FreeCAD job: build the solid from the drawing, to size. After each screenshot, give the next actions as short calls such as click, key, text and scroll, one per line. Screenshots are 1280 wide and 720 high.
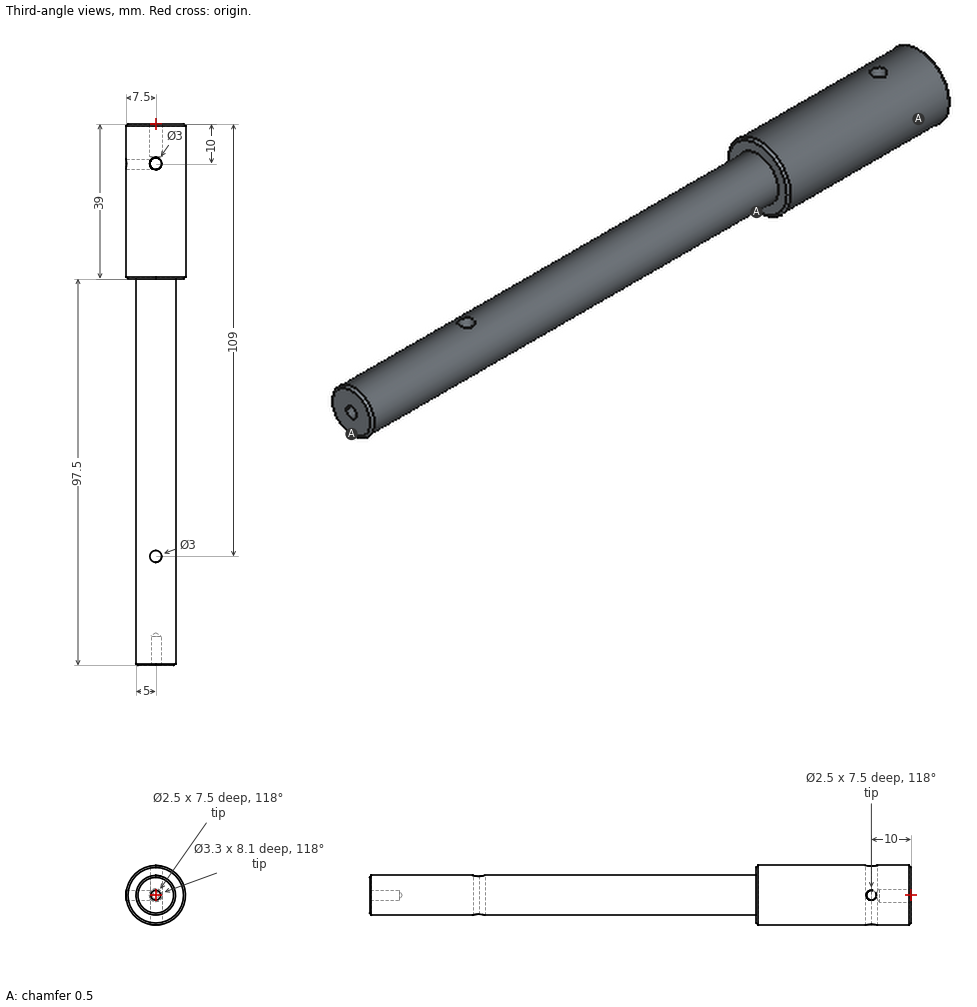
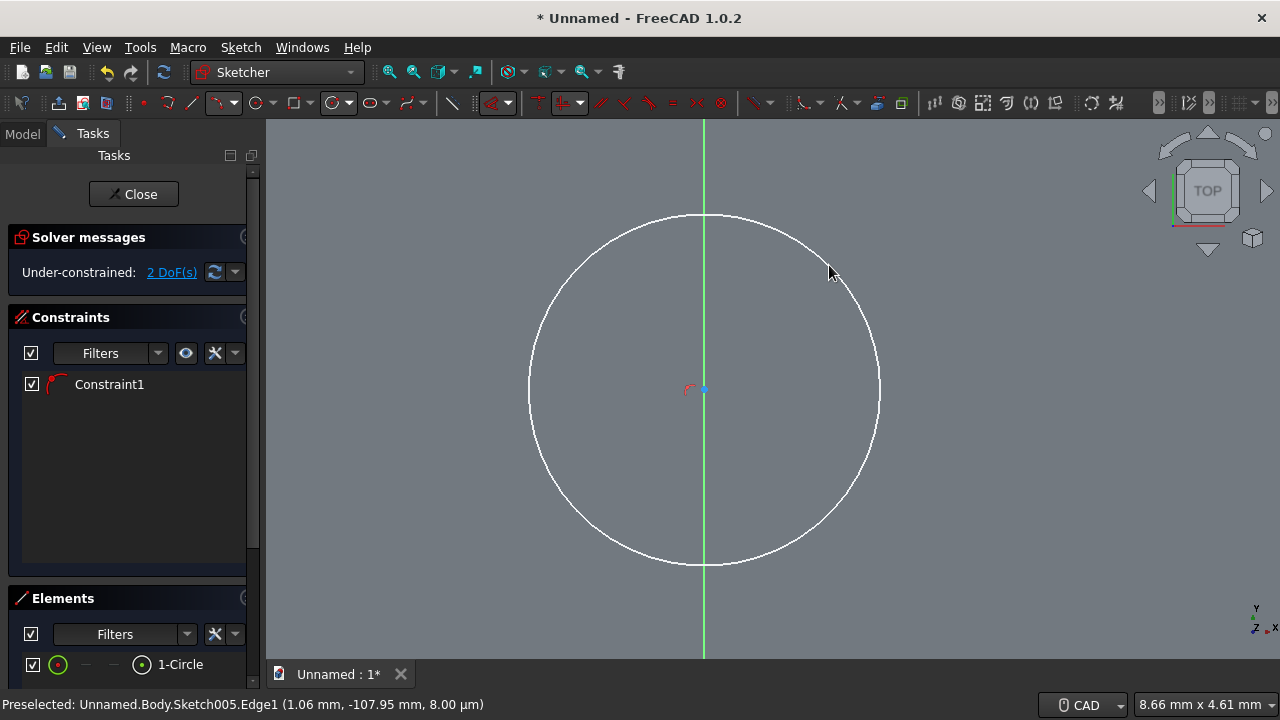
click(828, 265)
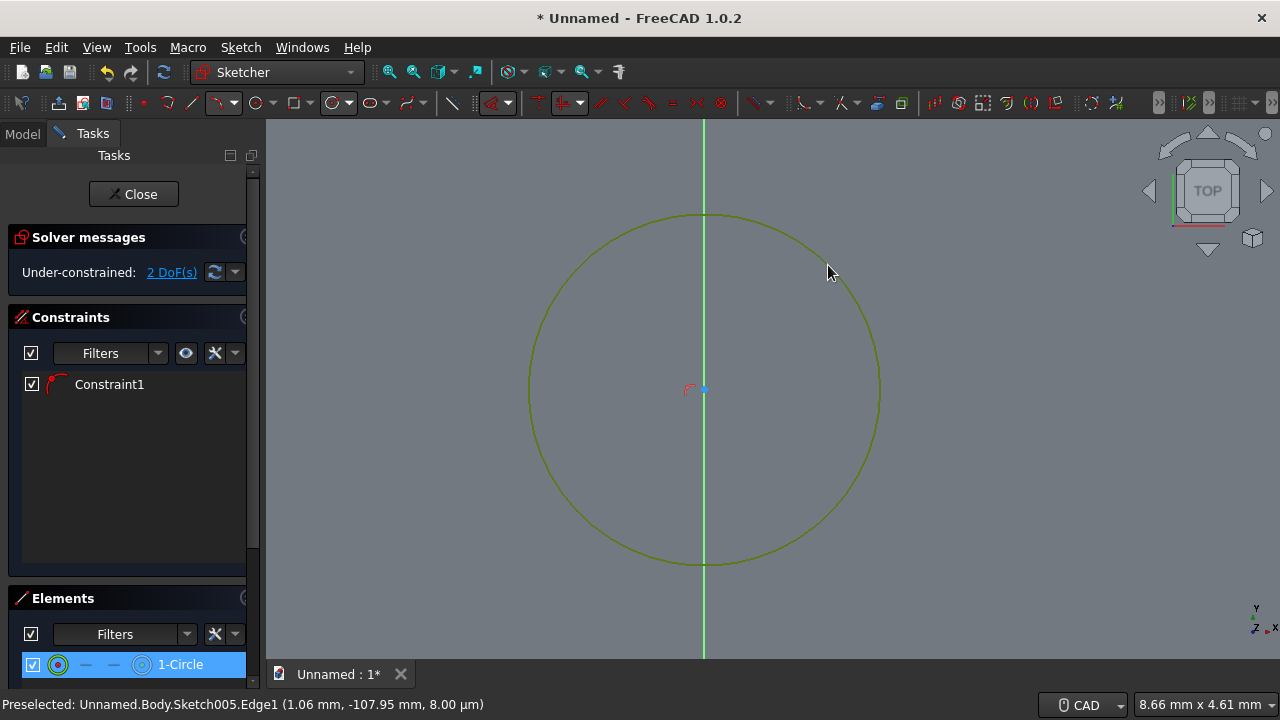
click(510, 104)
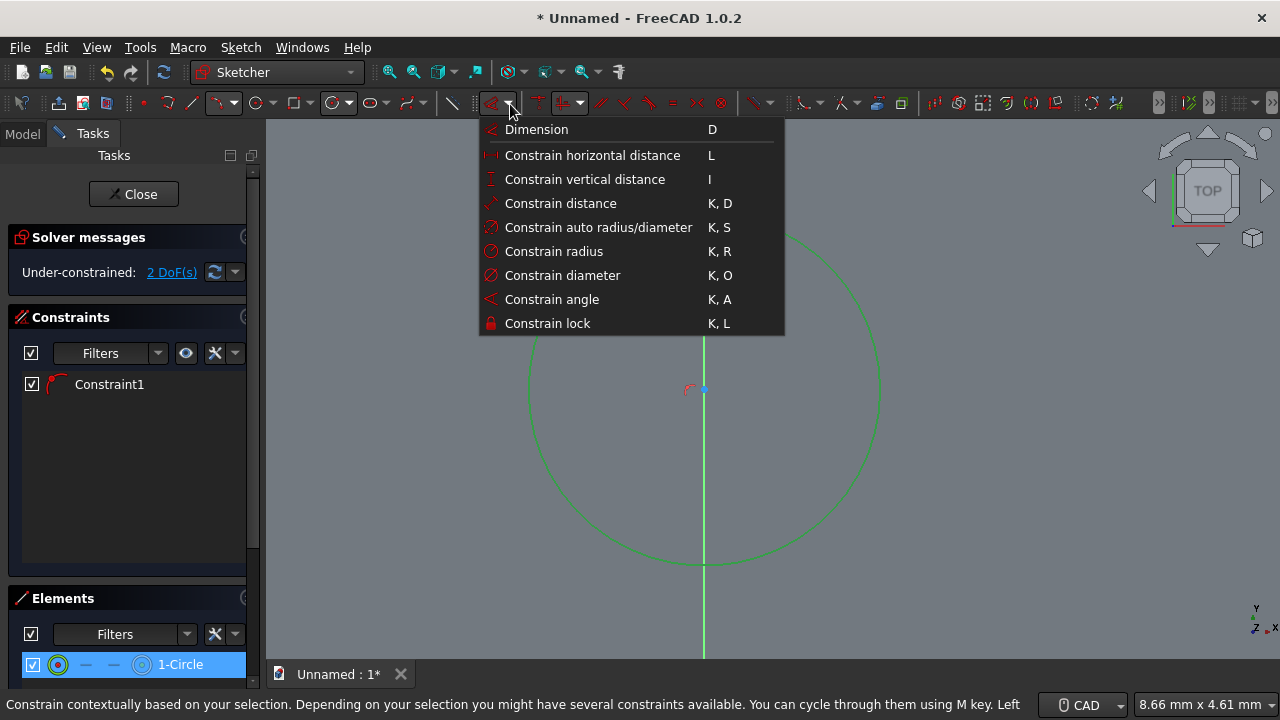
click(632, 275)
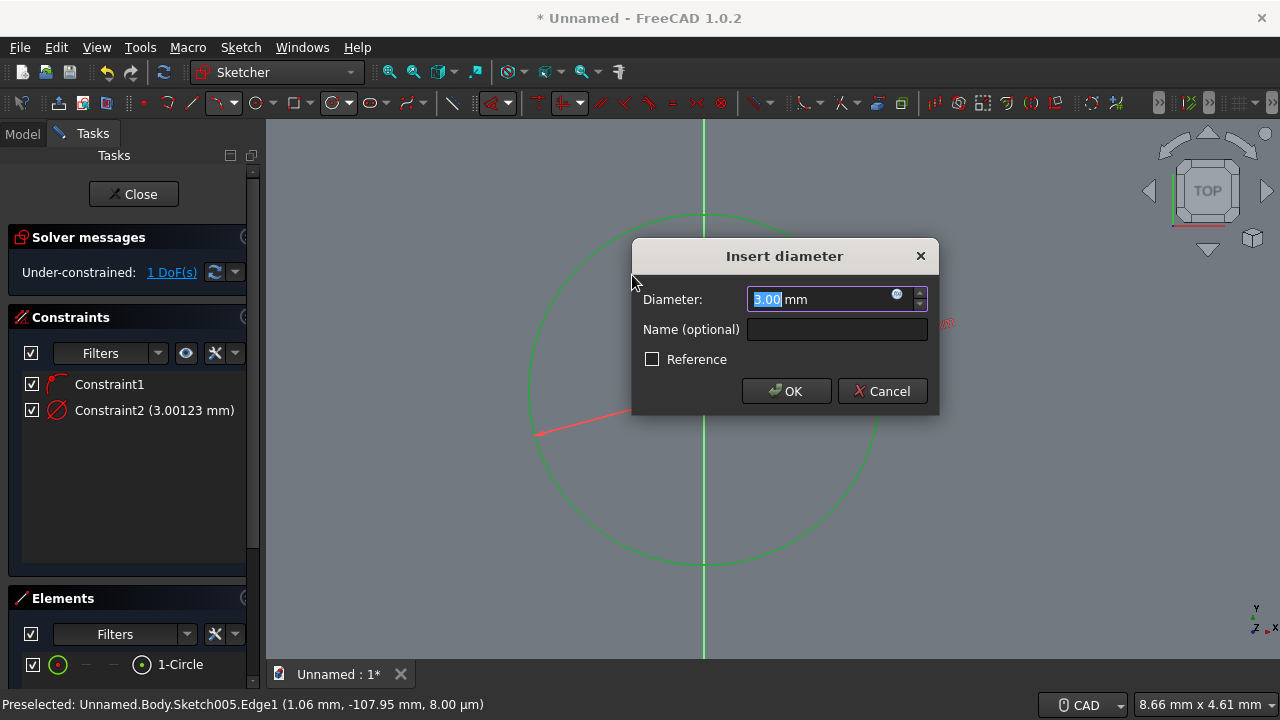
text(3)
key(Return)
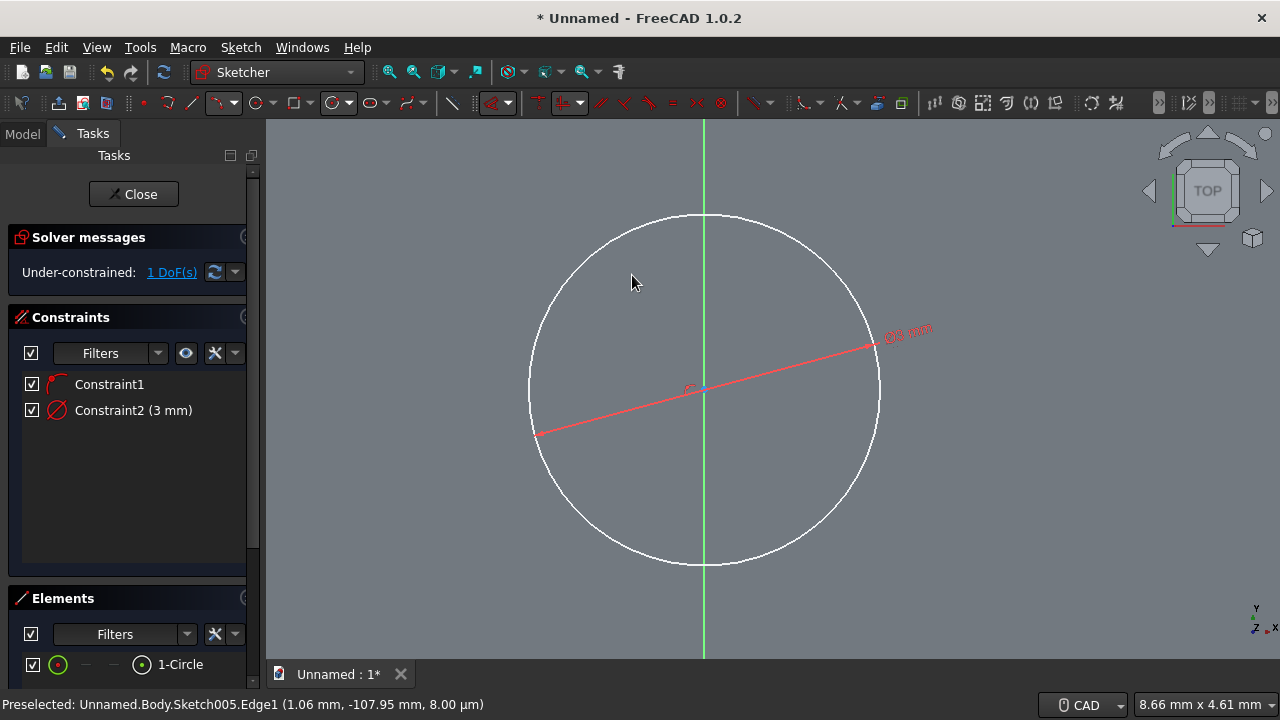
click(704, 390)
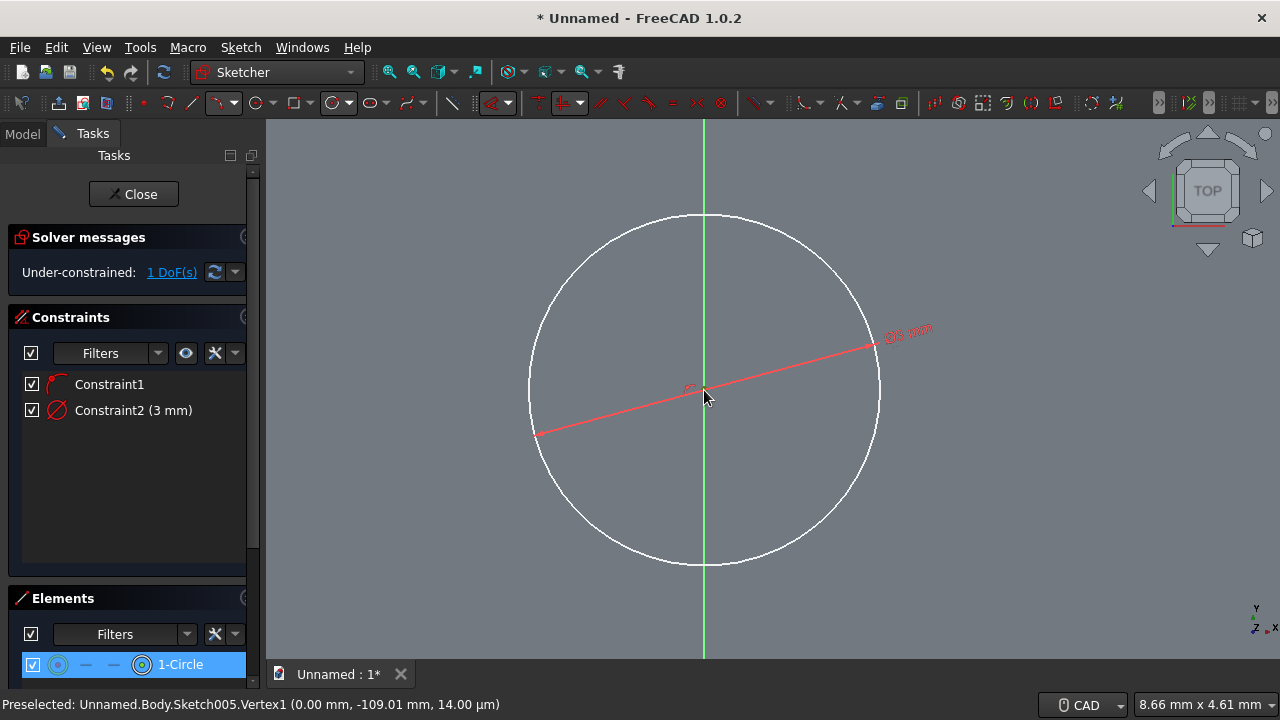
key(i)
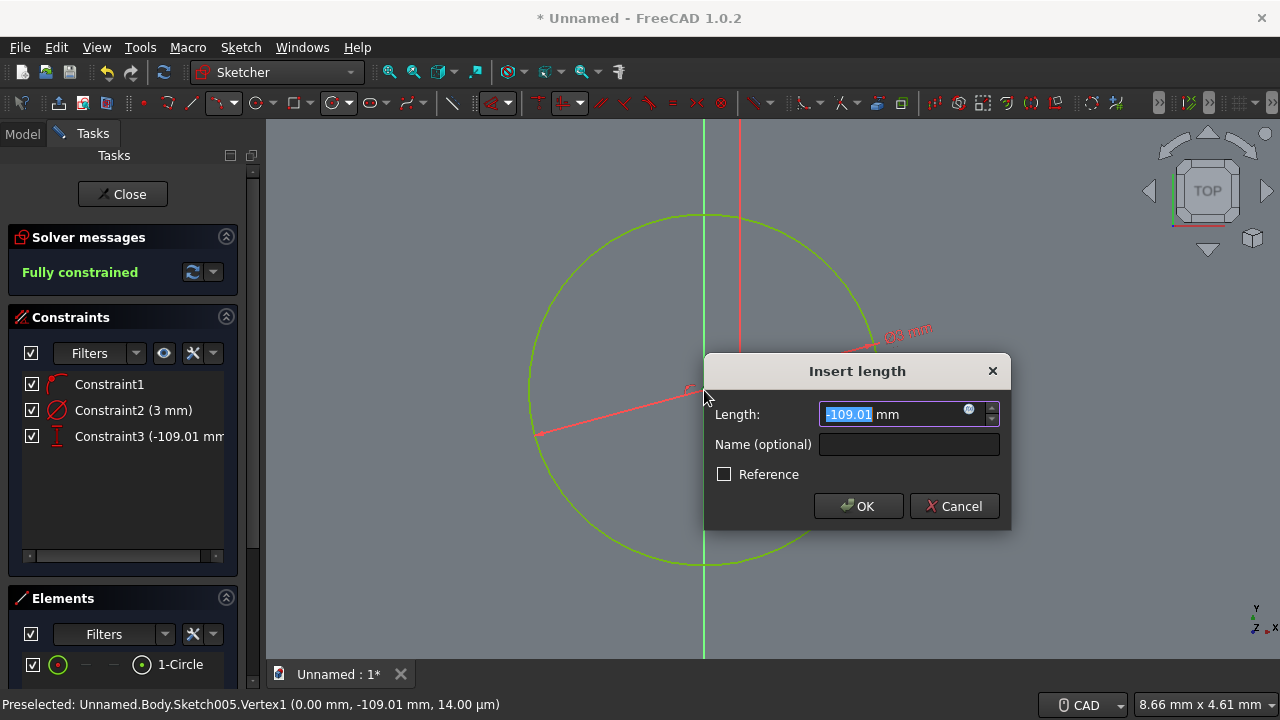
text(-109)
key(Return)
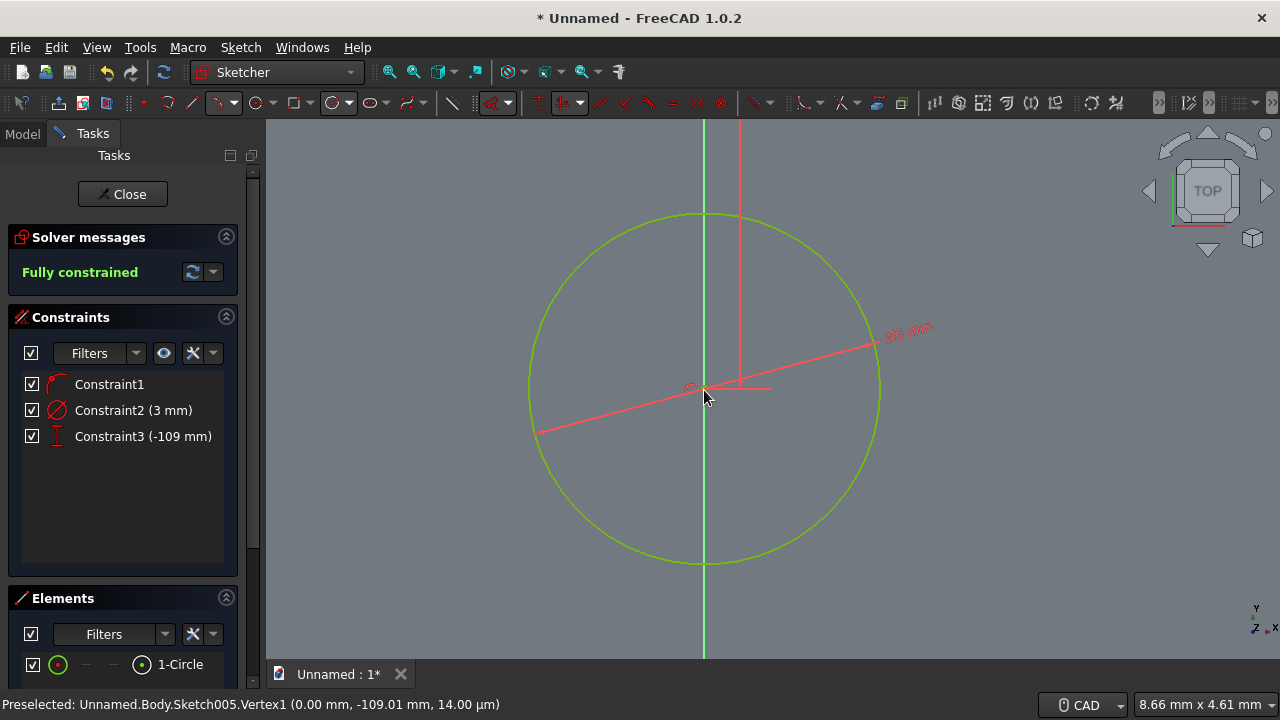
click(123, 194)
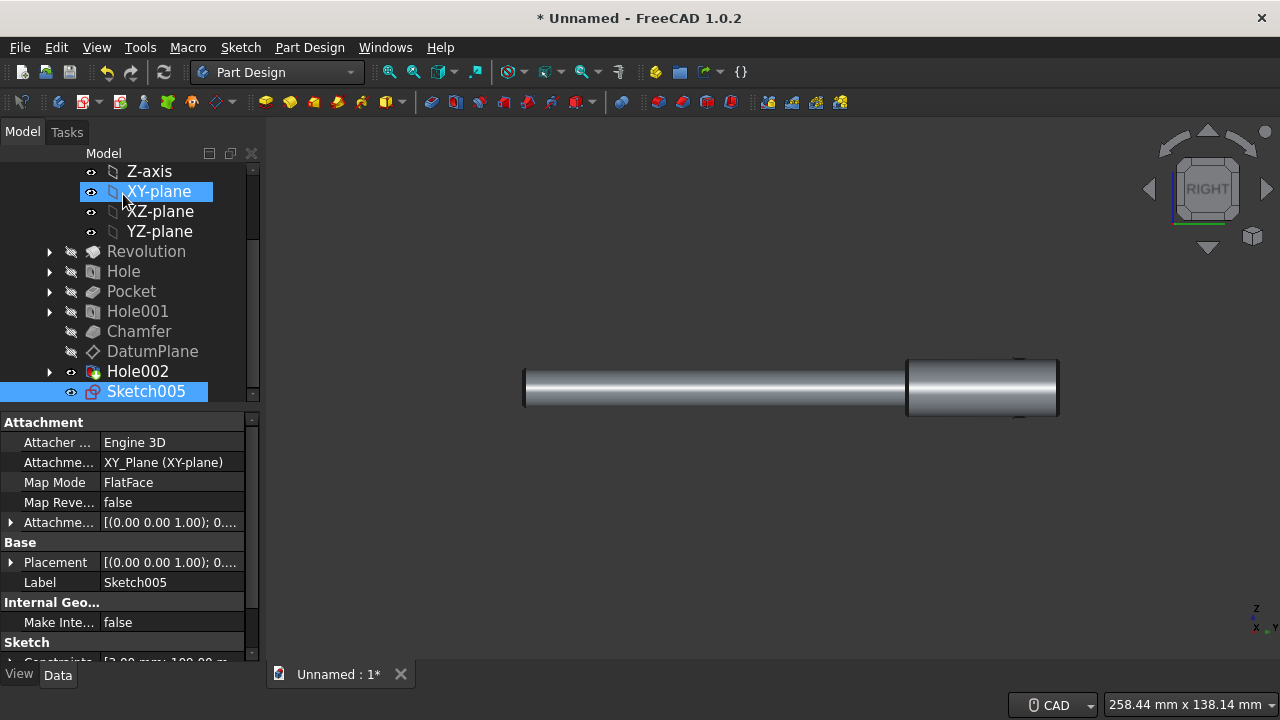
click(432, 102)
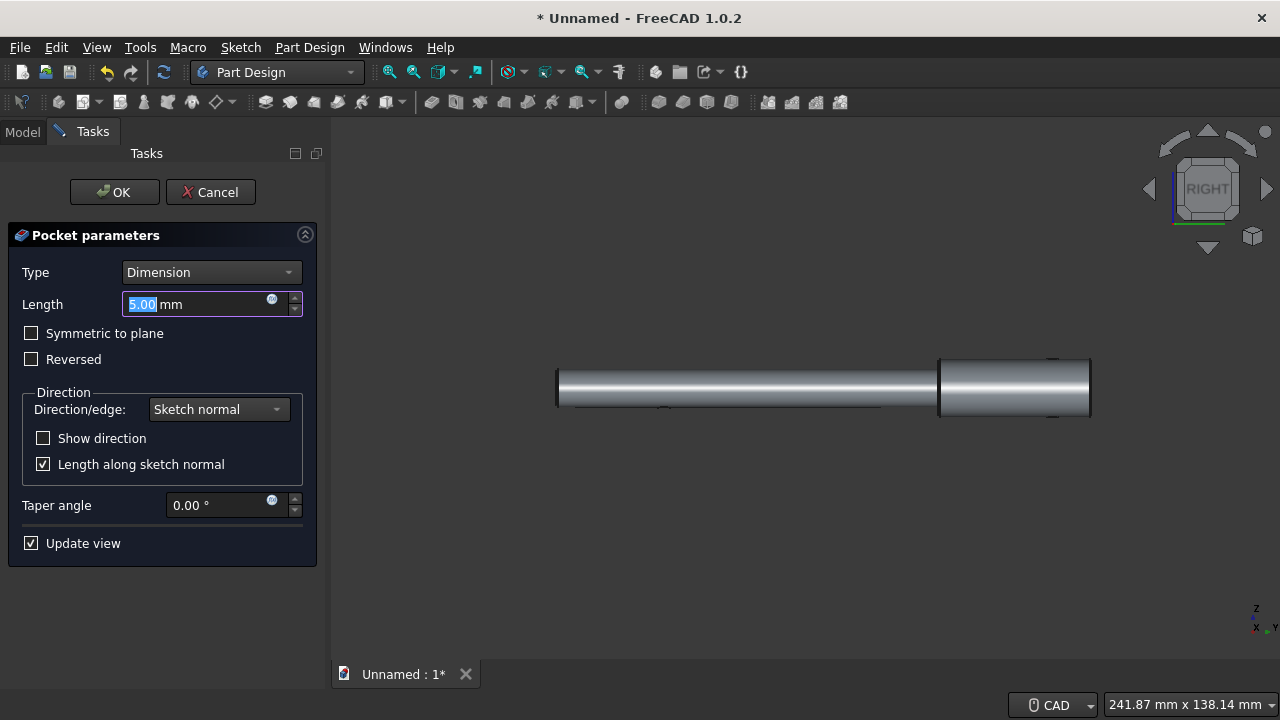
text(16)
key(Tab)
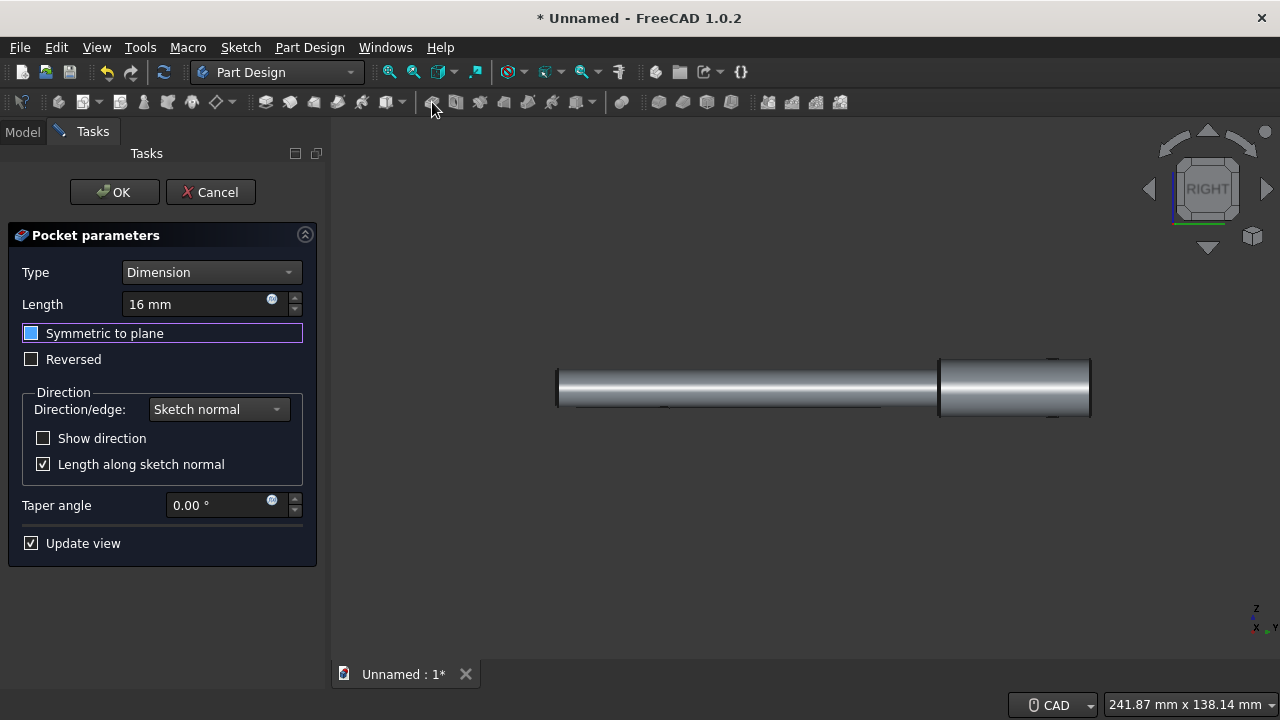
click(30, 333)